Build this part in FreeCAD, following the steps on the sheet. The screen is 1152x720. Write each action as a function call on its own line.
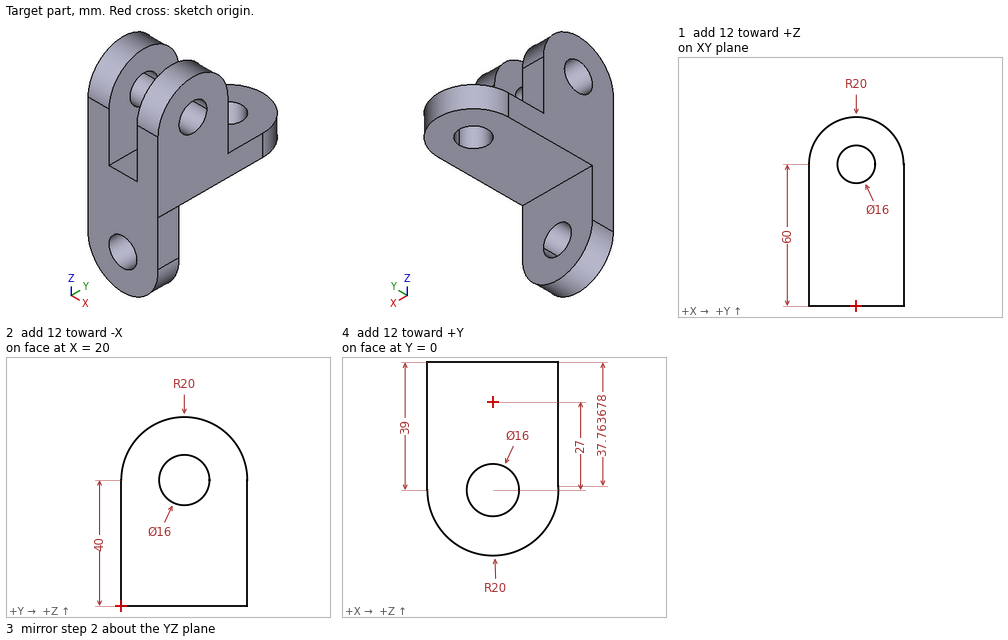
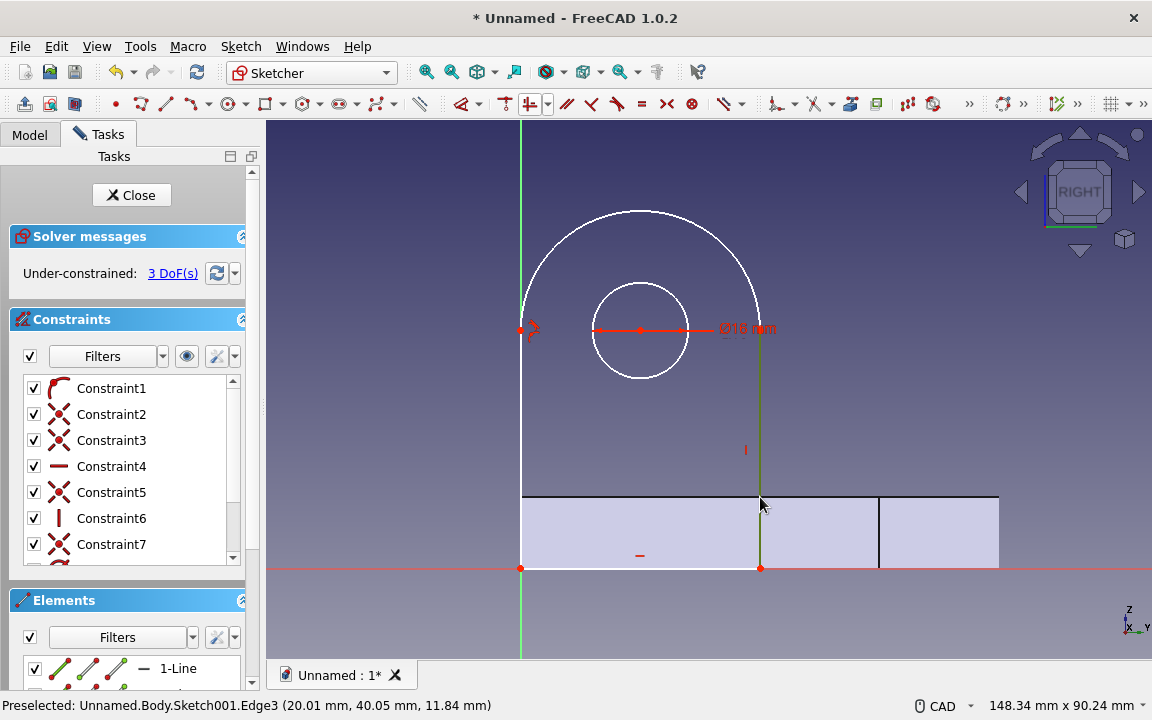
click(711, 234)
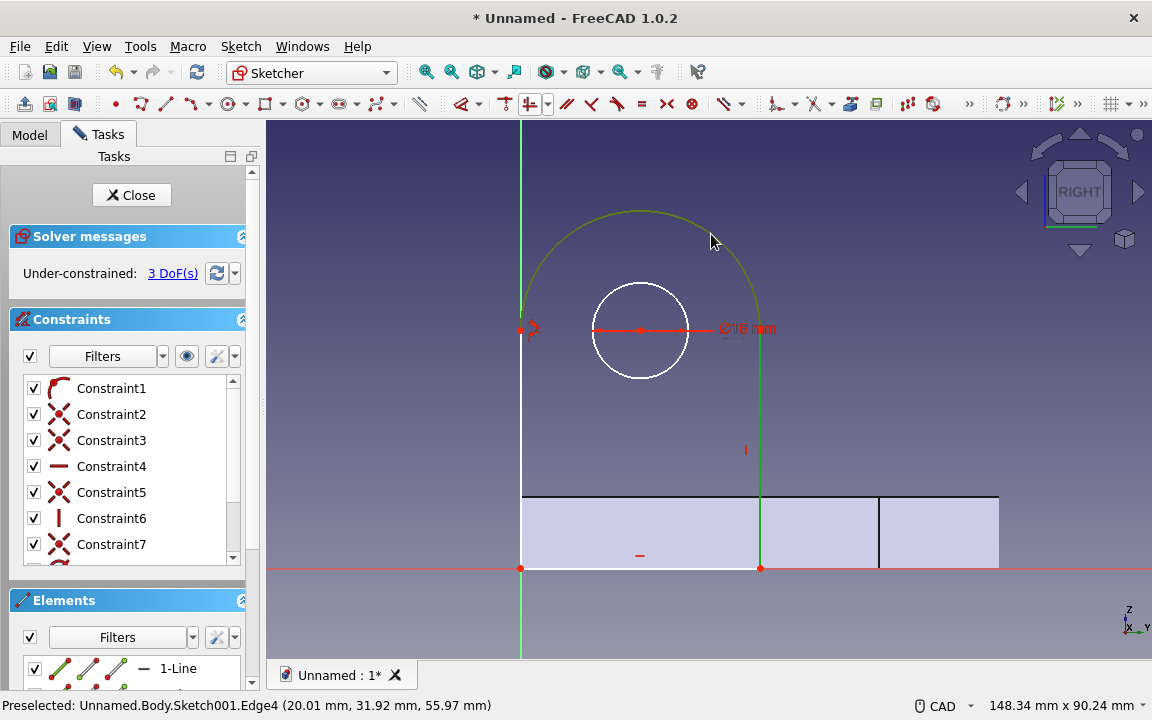
key(t)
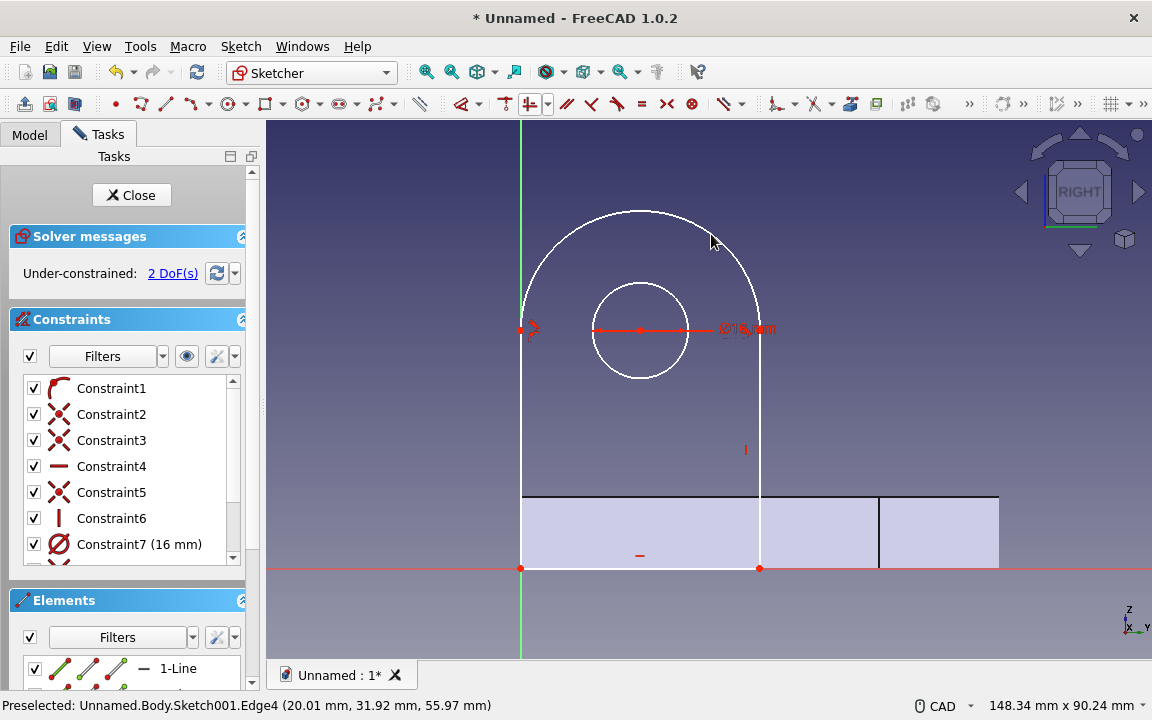
click(460, 104)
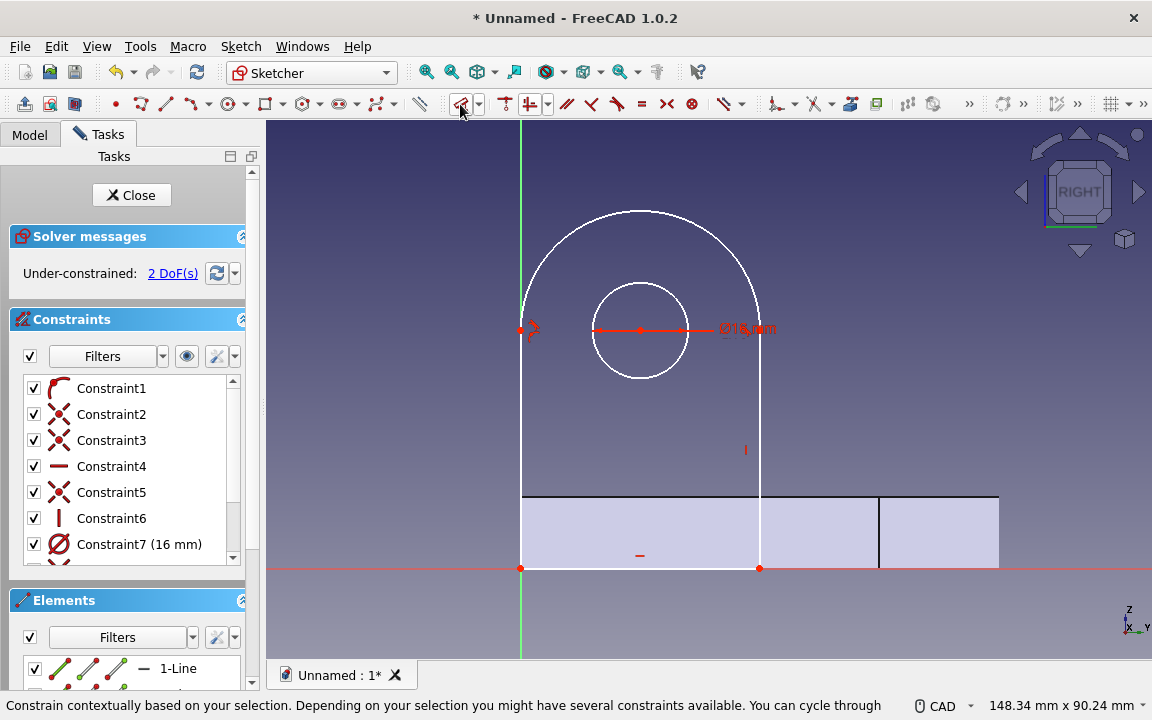
click(711, 234)
click(730, 208)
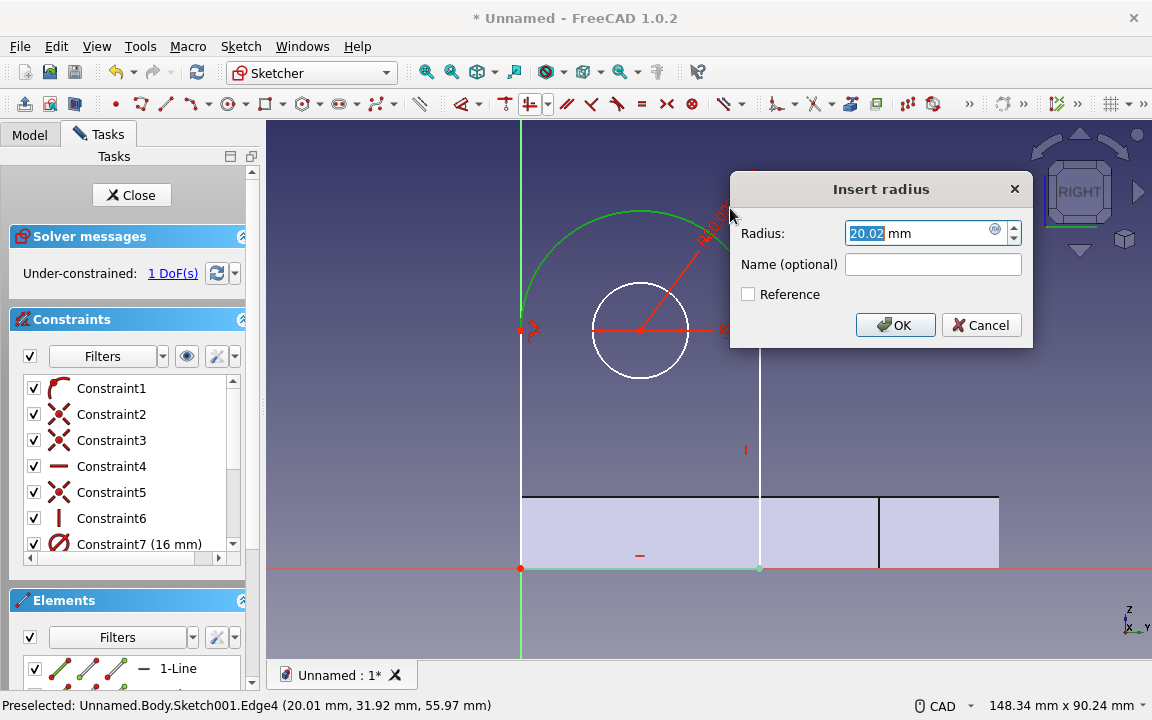
text(20)
key(Return)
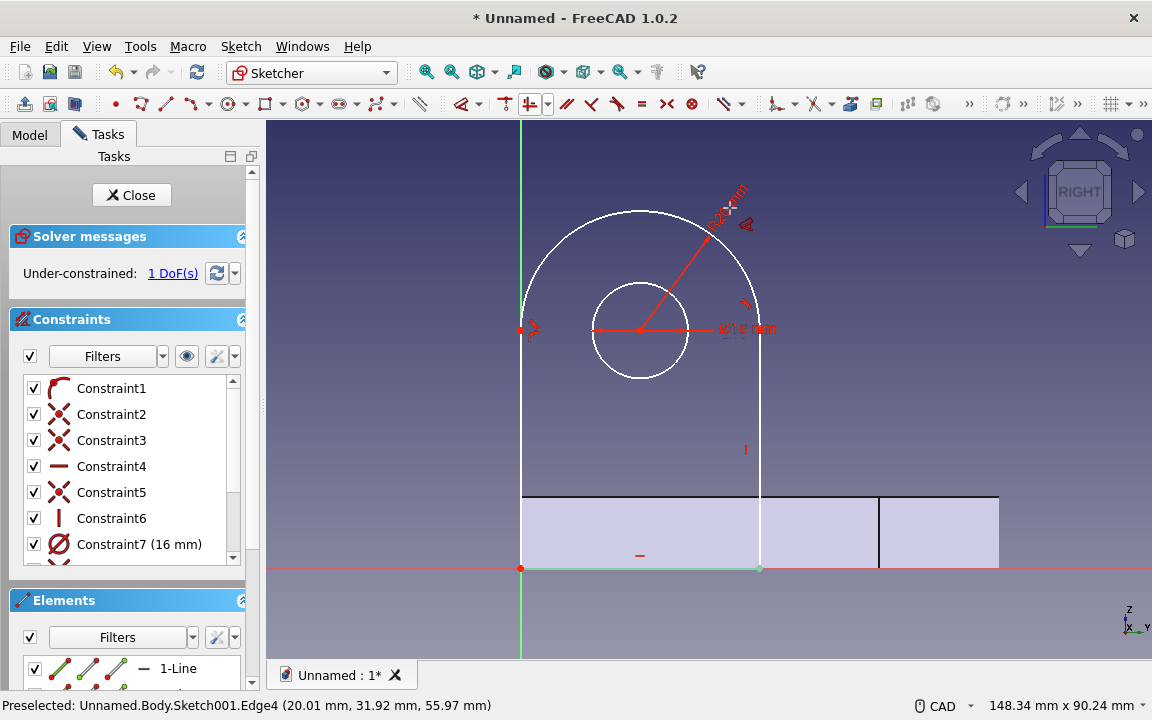
click(521, 402)
click(487, 450)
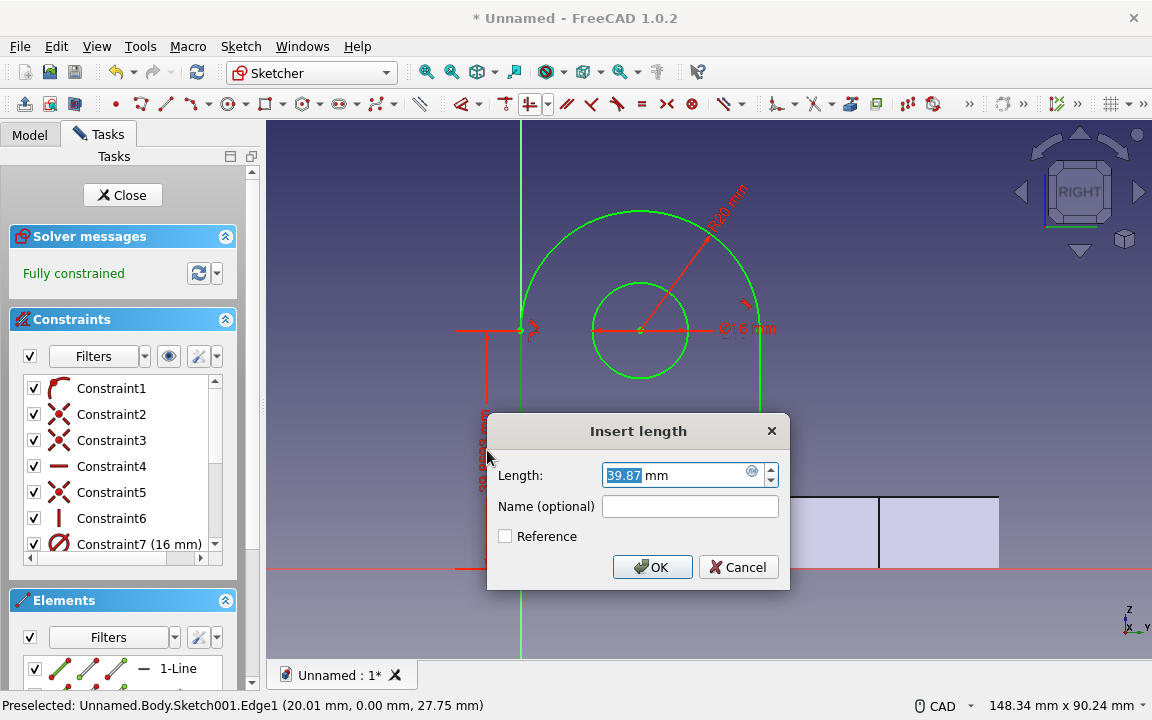
text(40)
key(Return)
key(Escape)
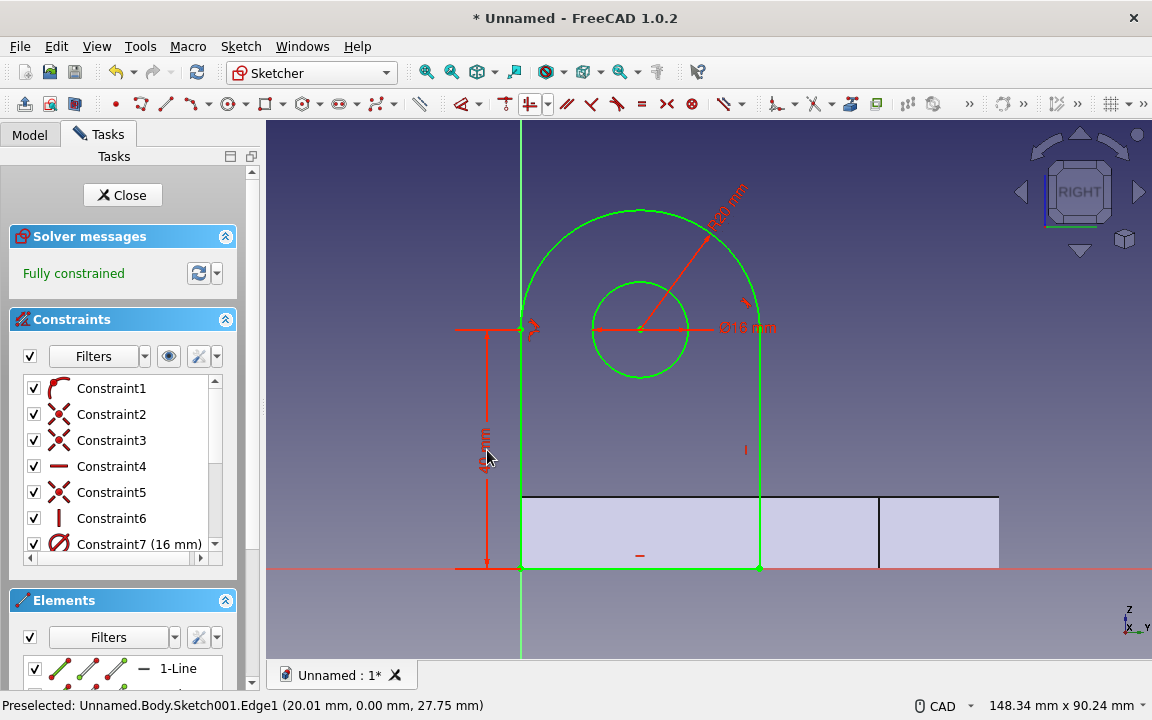
click(123, 195)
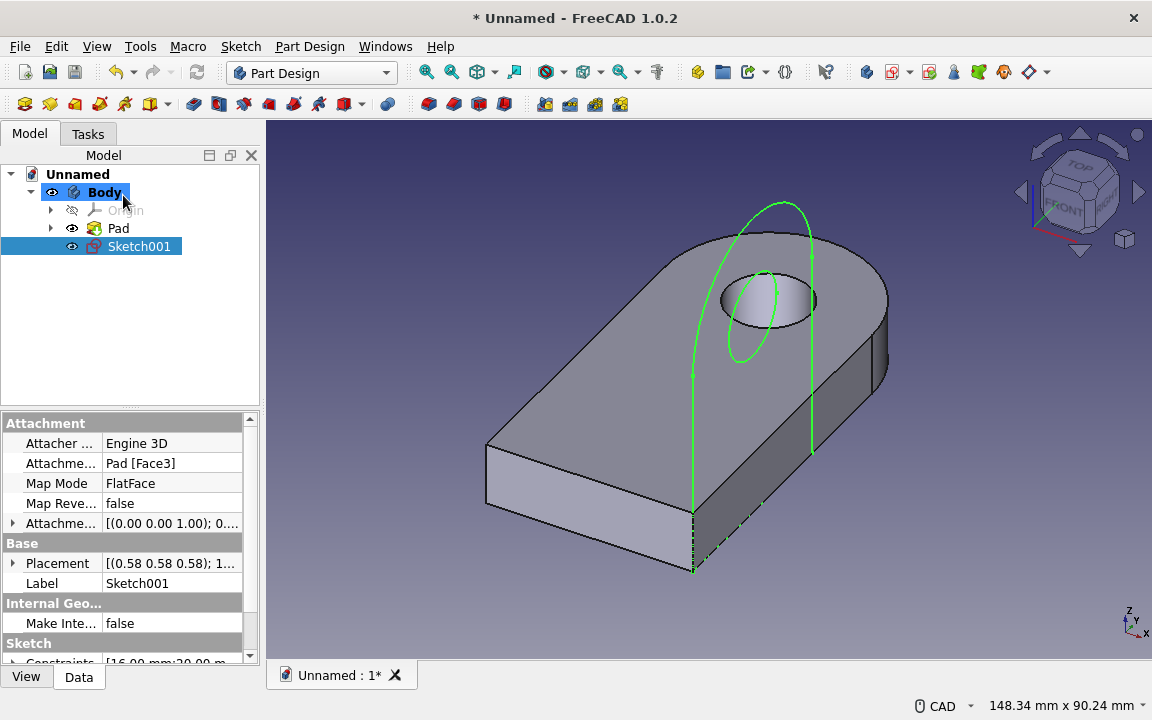
click(25, 104)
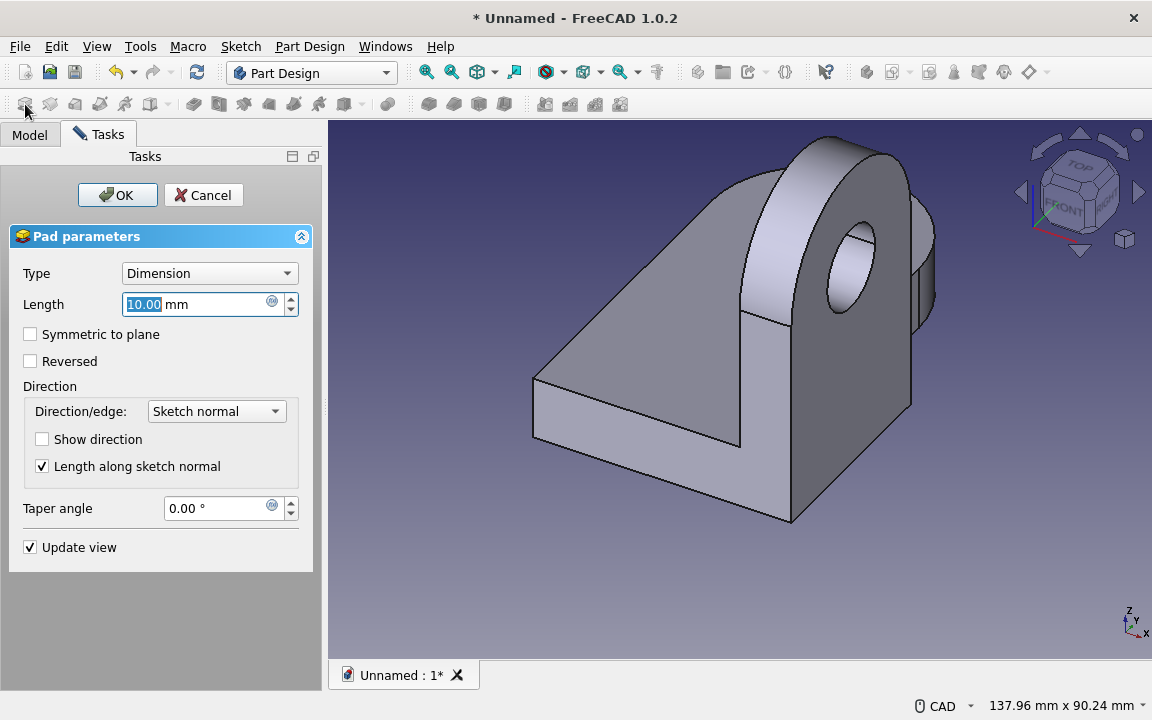
text(12)
key(Tab)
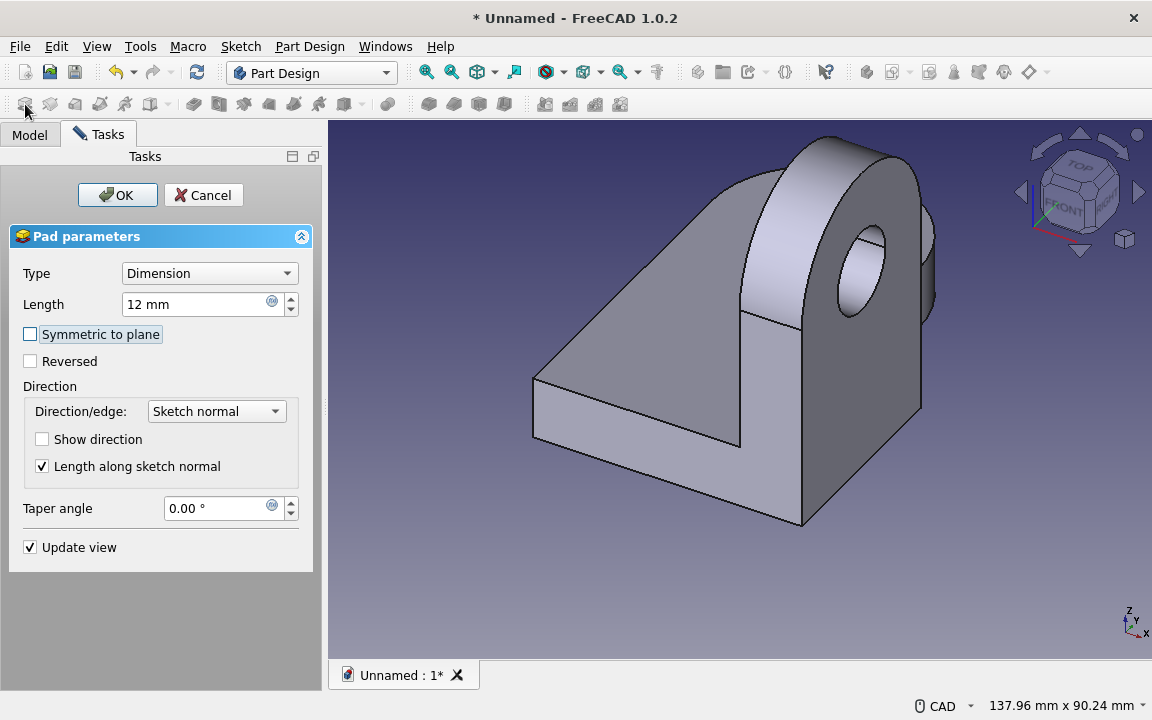
click(31, 361)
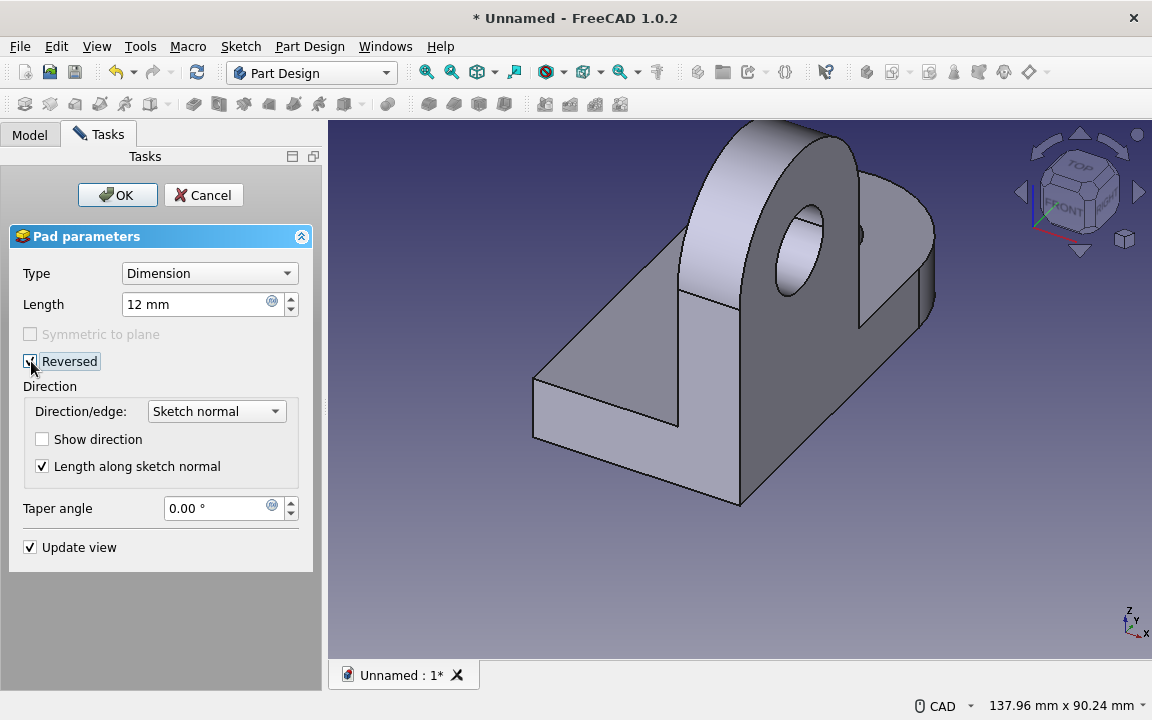
click(118, 195)